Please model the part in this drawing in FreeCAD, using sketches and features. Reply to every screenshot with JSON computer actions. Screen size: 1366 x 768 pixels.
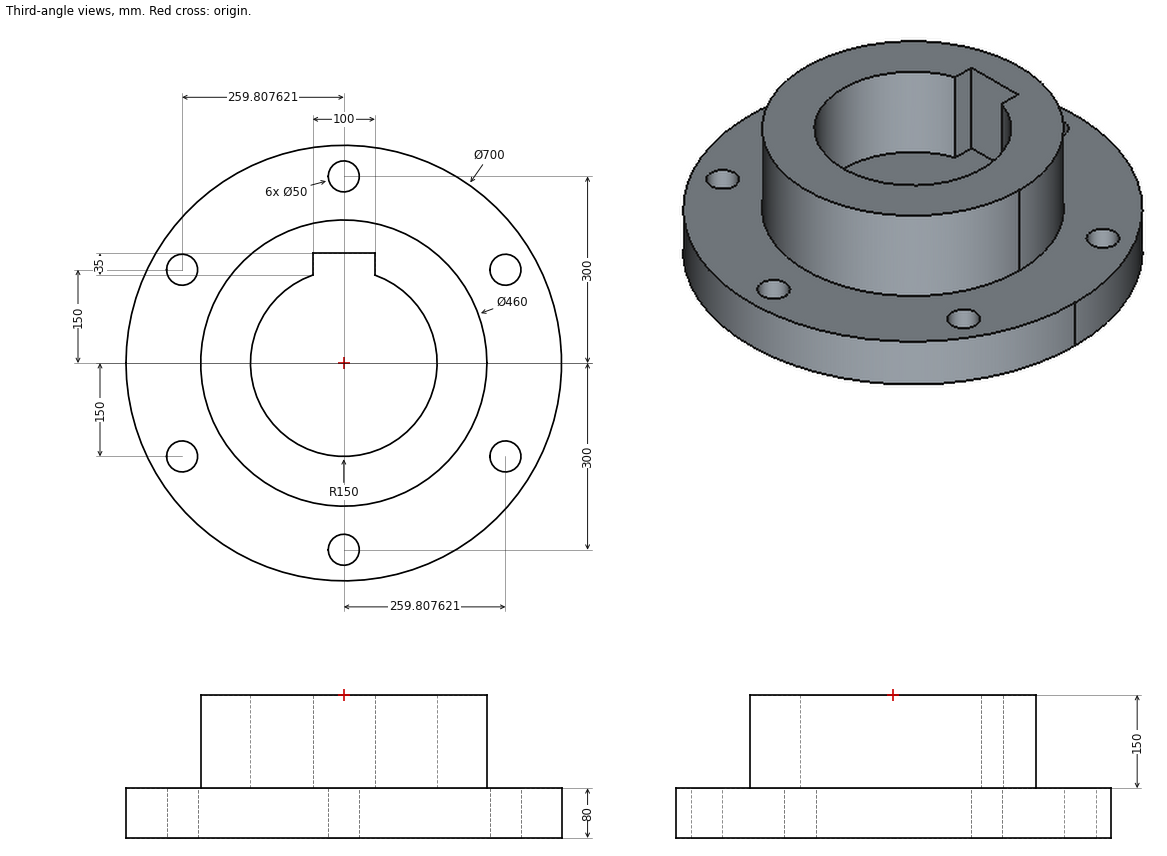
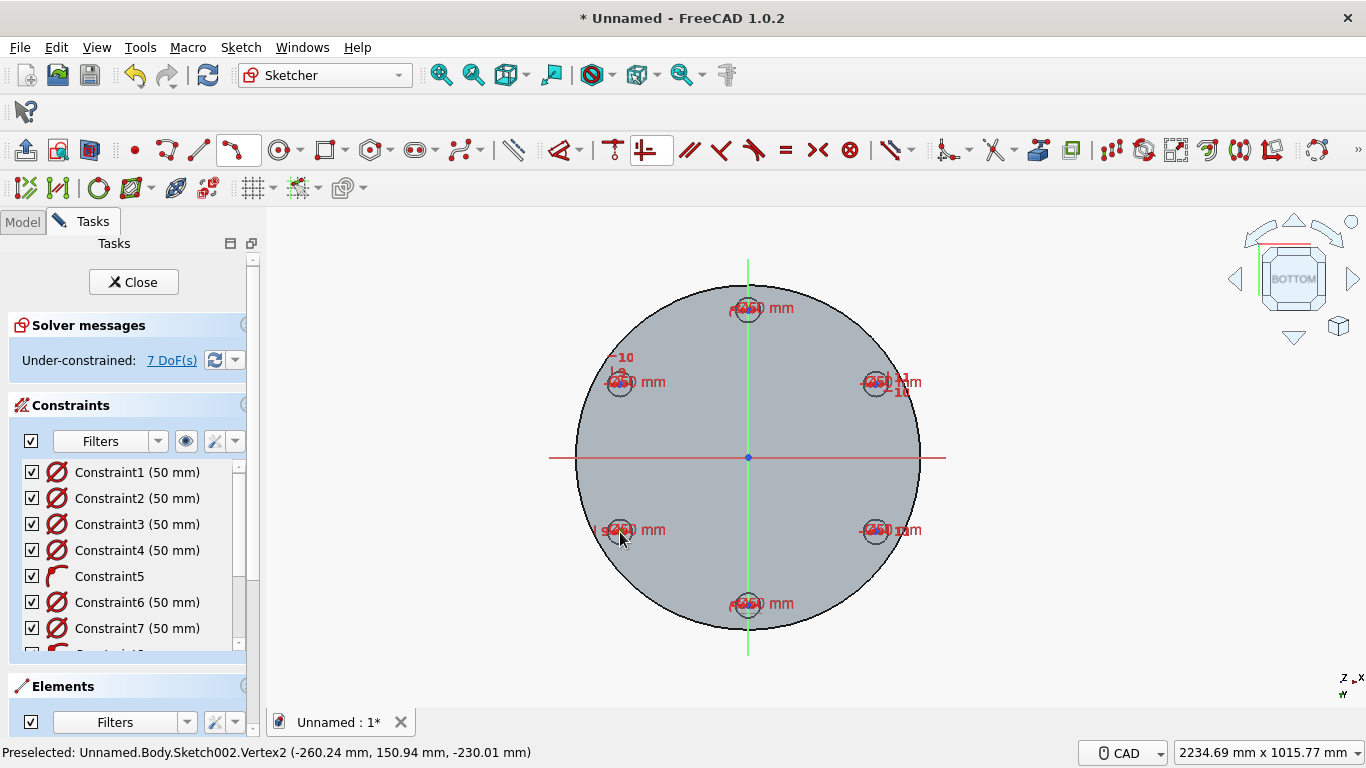
{"action": "left_click", "coordinate": [876, 532]}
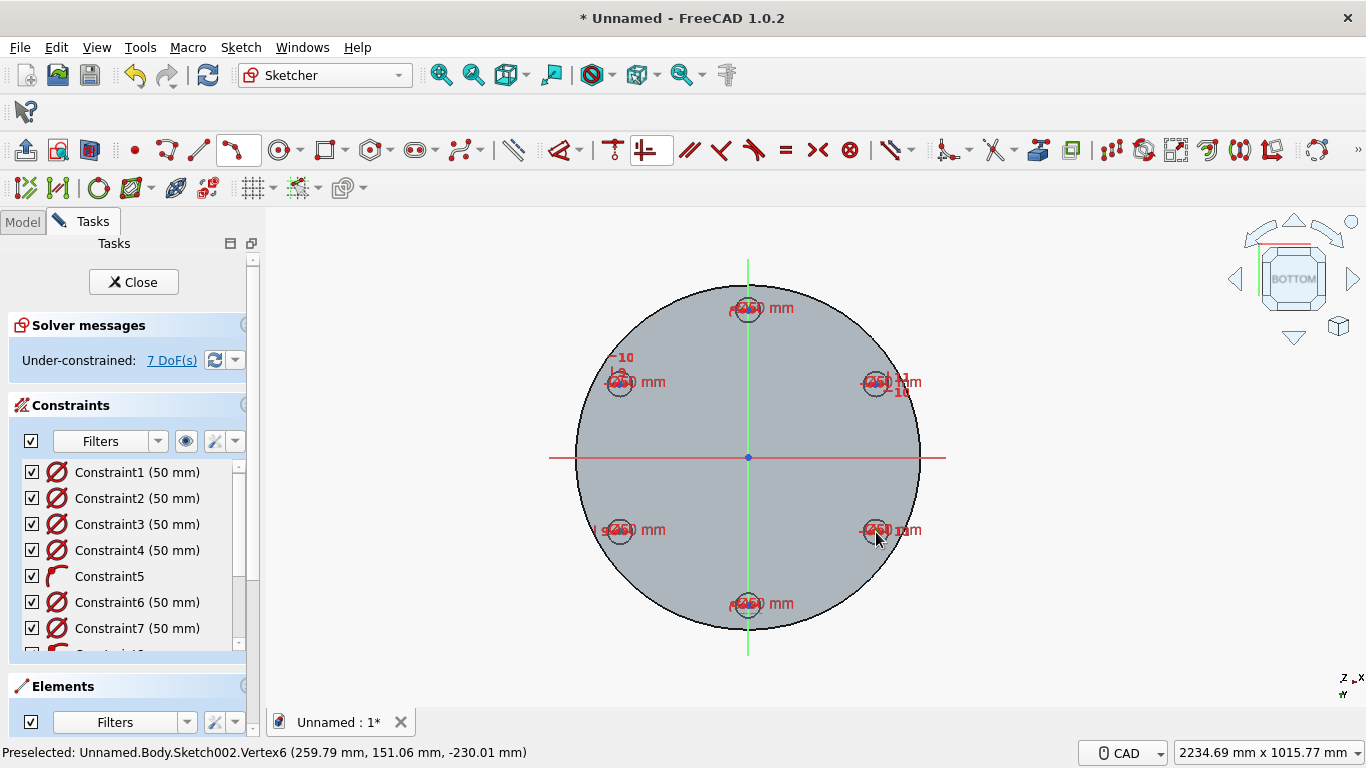
{"action": "key", "text": "h"}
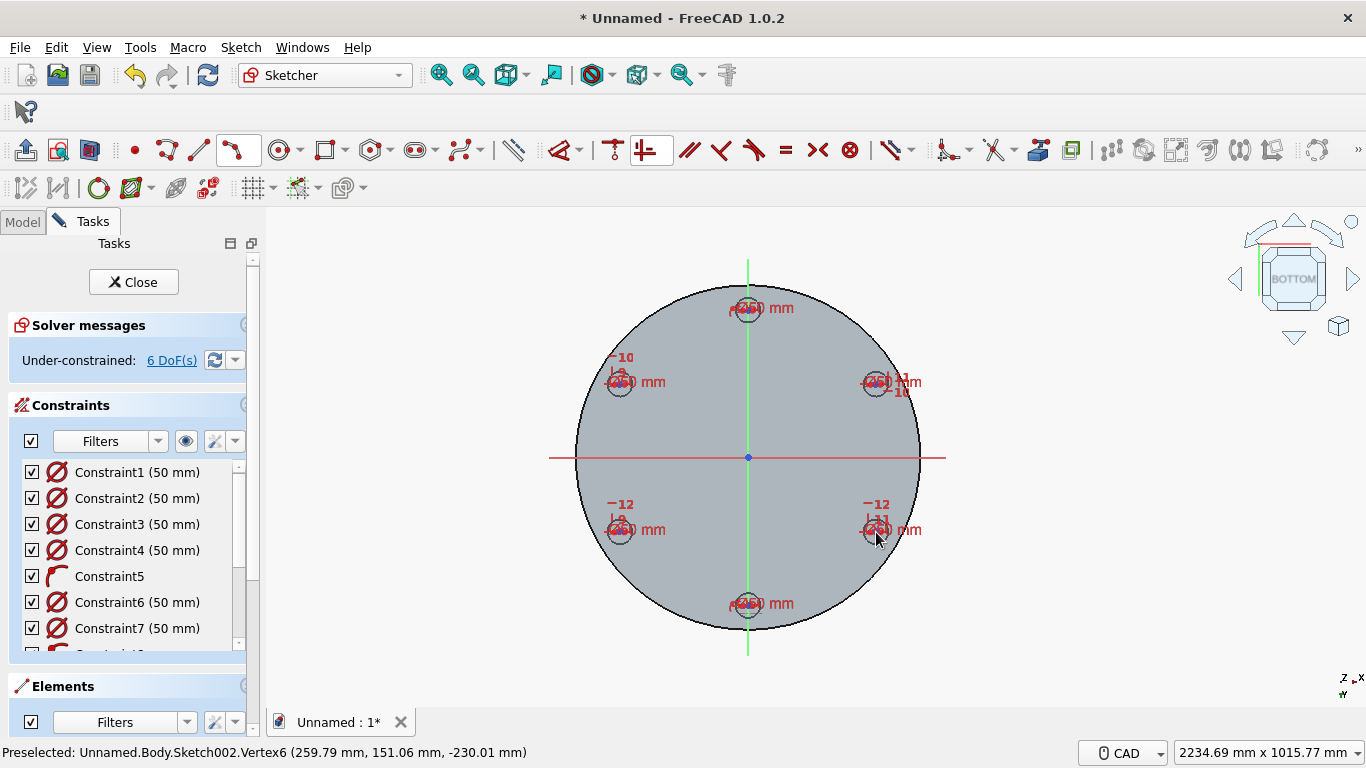
{"action": "key", "text": "d"}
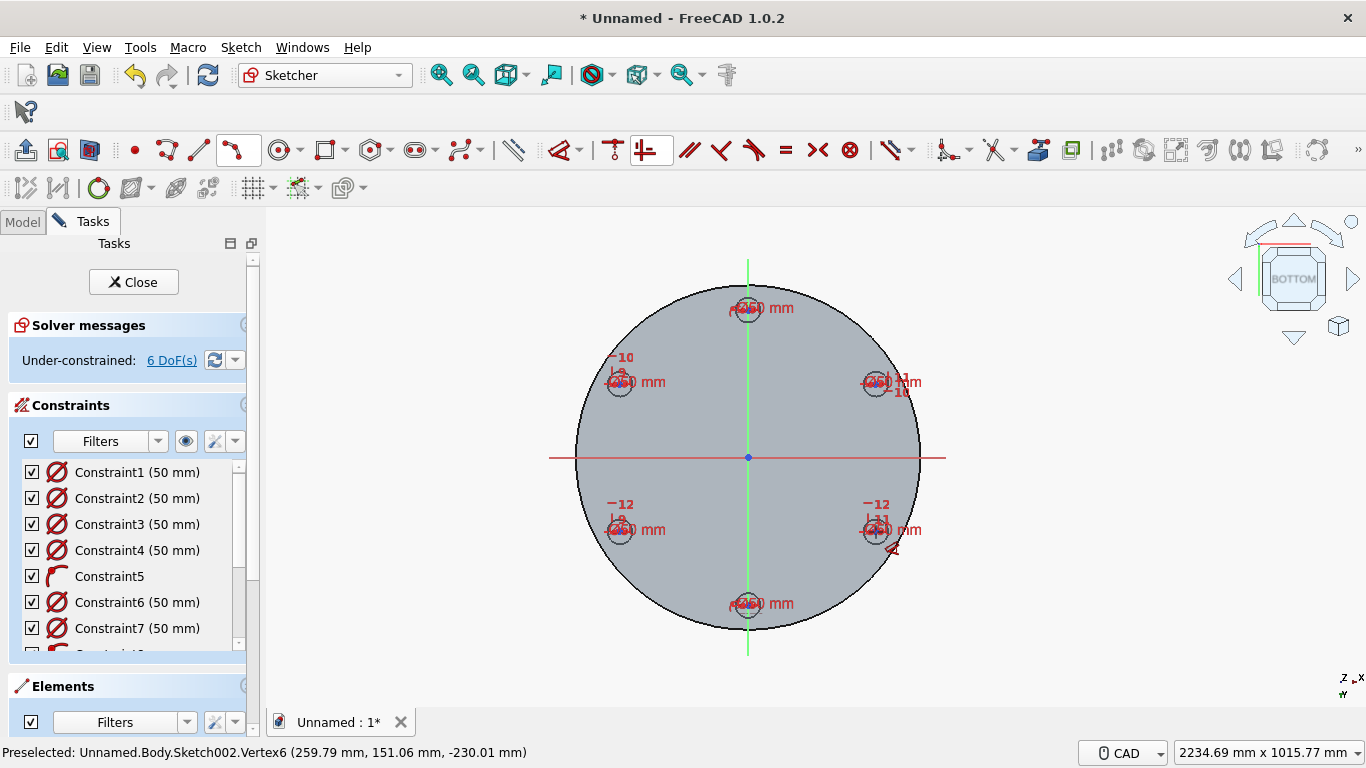
{"action": "left_click", "coordinate": [748, 606]}
{"action": "left_click", "coordinate": [782, 532]}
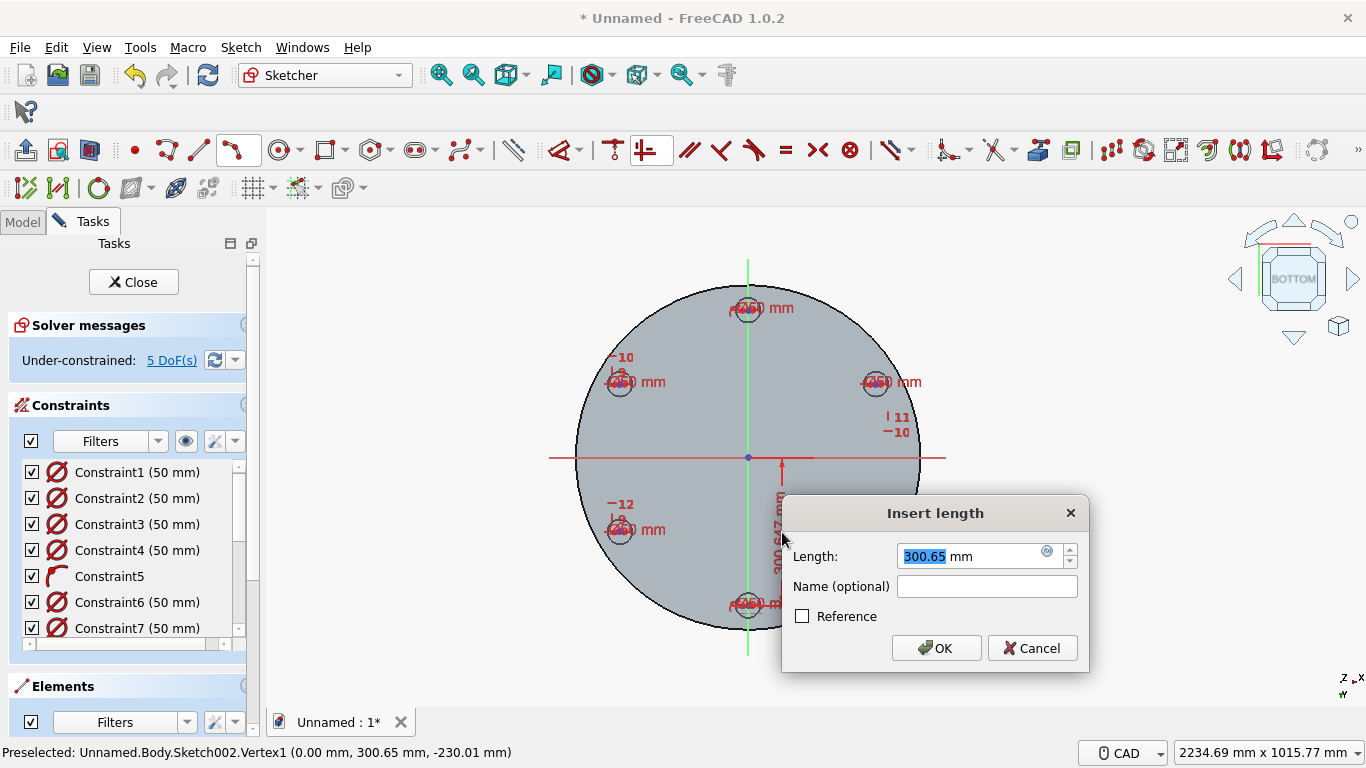
{"action": "type", "text": "300"}
{"action": "key", "text": "Return"}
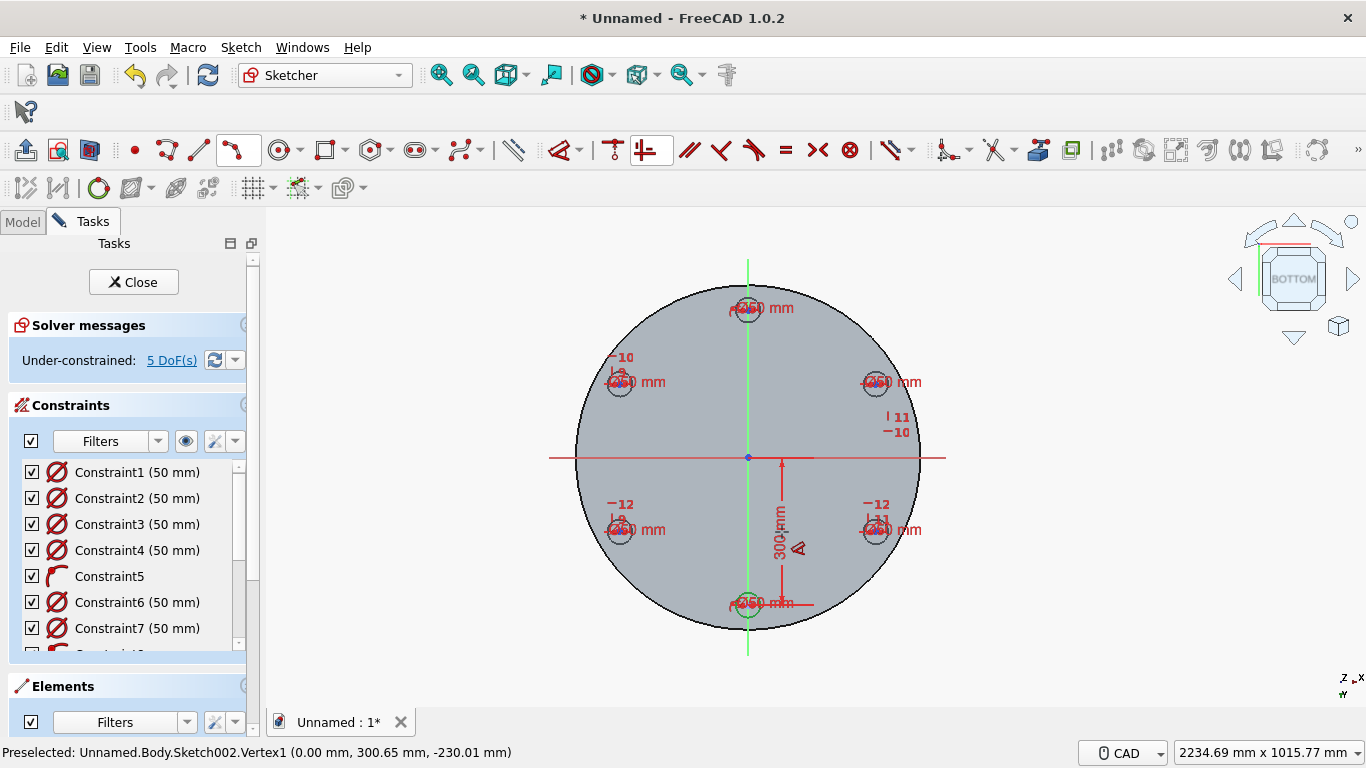
{"action": "left_click", "coordinate": [620, 532]}
{"action": "left_click", "coordinate": [586, 495]}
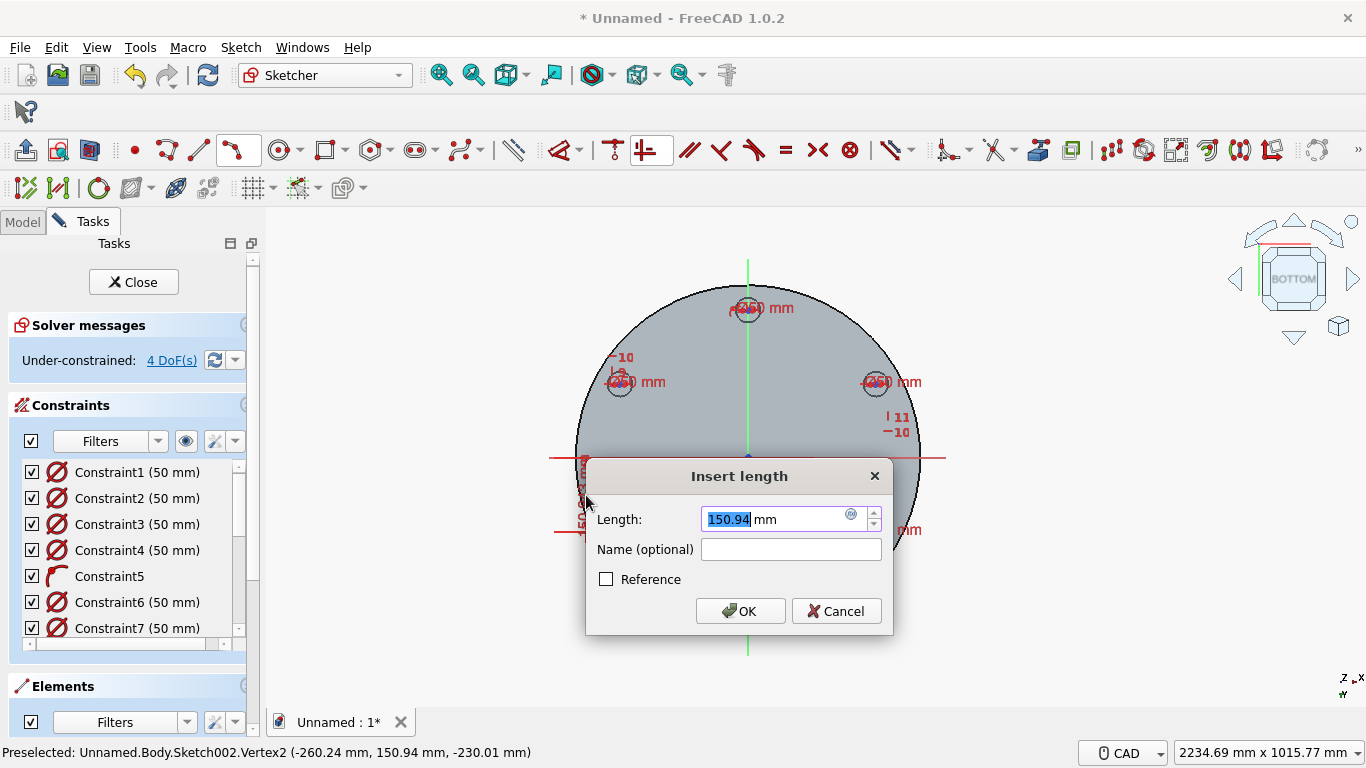
{"action": "type", "text": "150"}
{"action": "key", "text": "Return"}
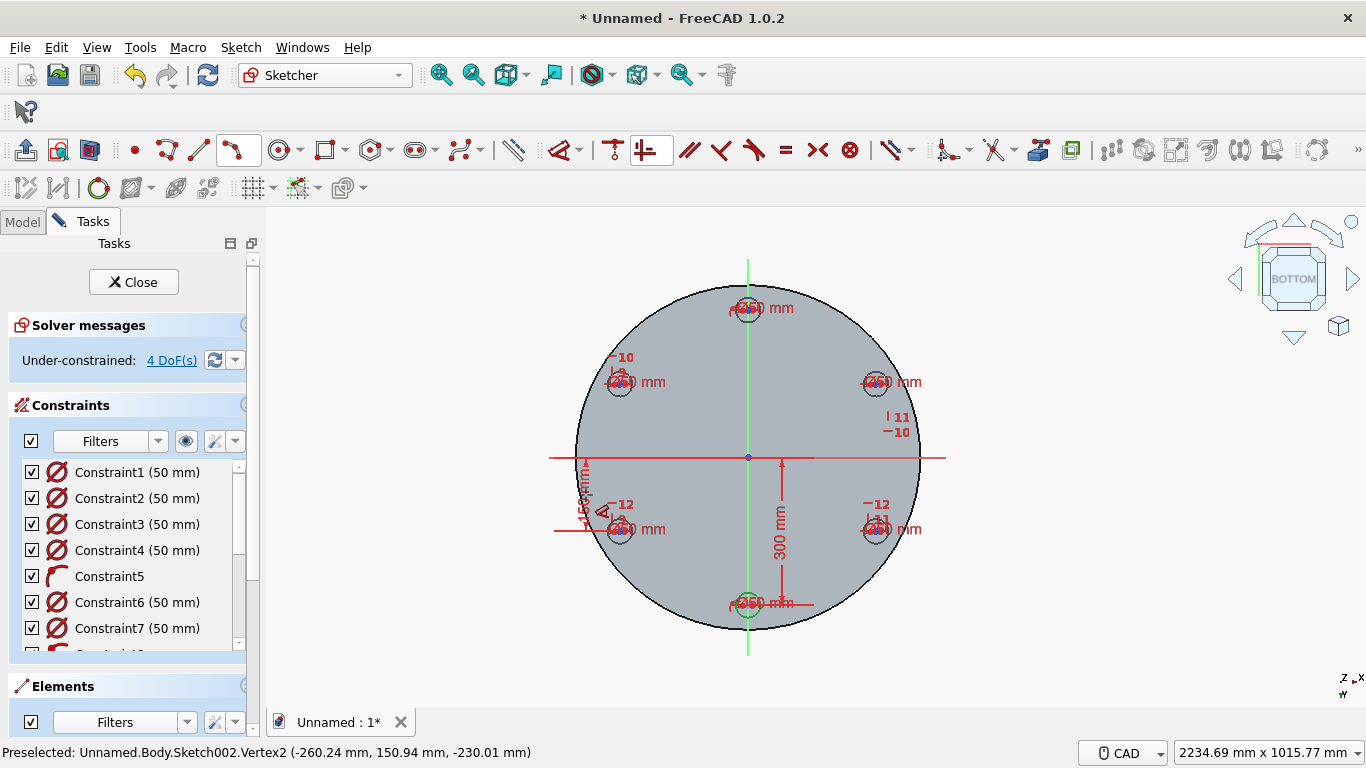
{"action": "left_click", "coordinate": [620, 384]}
{"action": "left_click", "coordinate": [586, 421]}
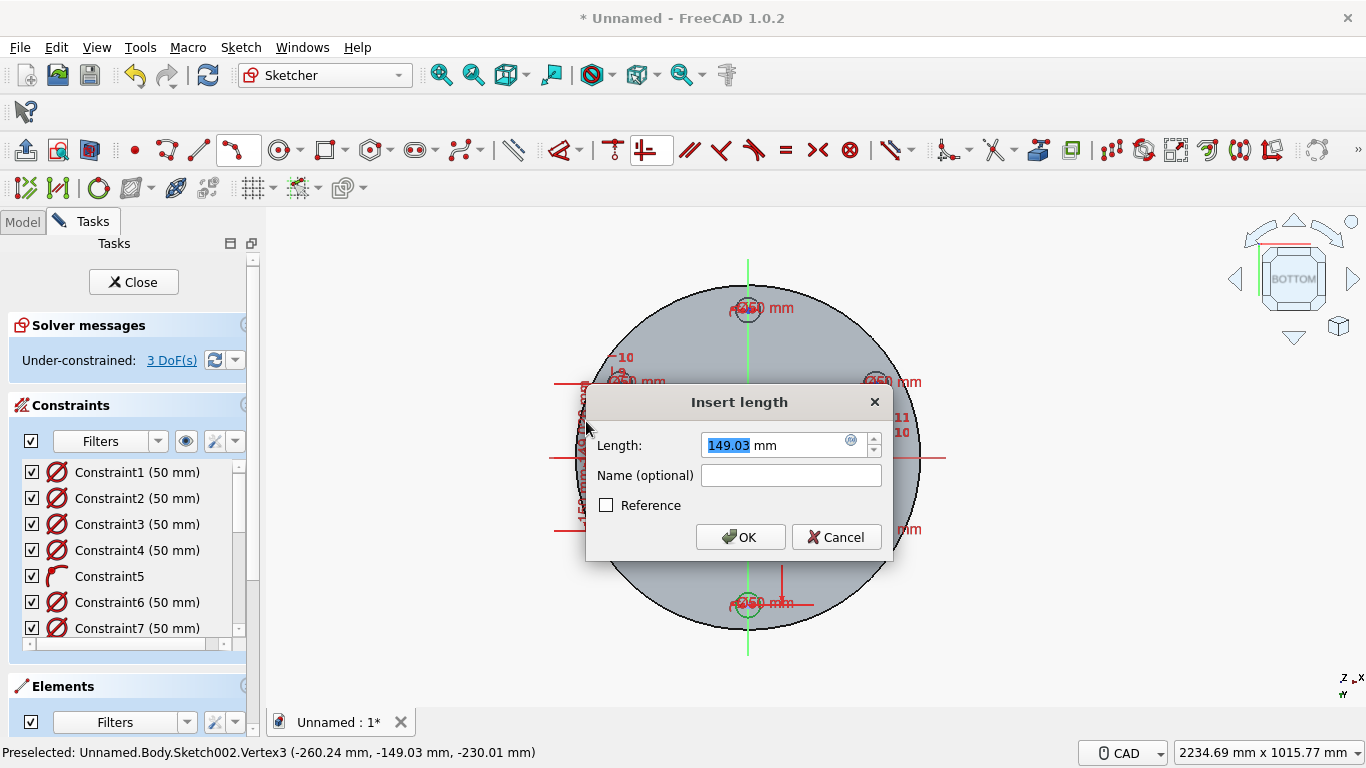
{"action": "type", "text": "150"}
{"action": "key", "text": "Return"}